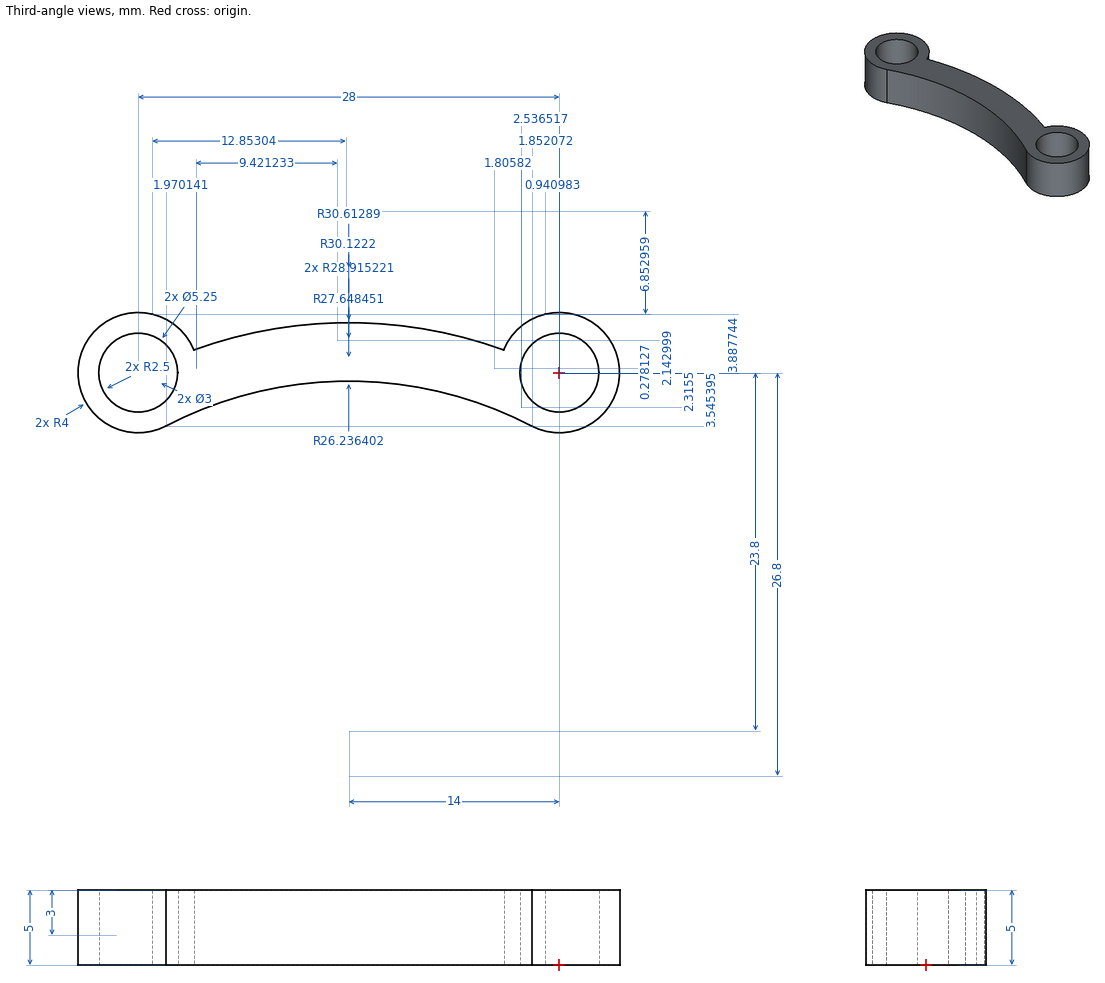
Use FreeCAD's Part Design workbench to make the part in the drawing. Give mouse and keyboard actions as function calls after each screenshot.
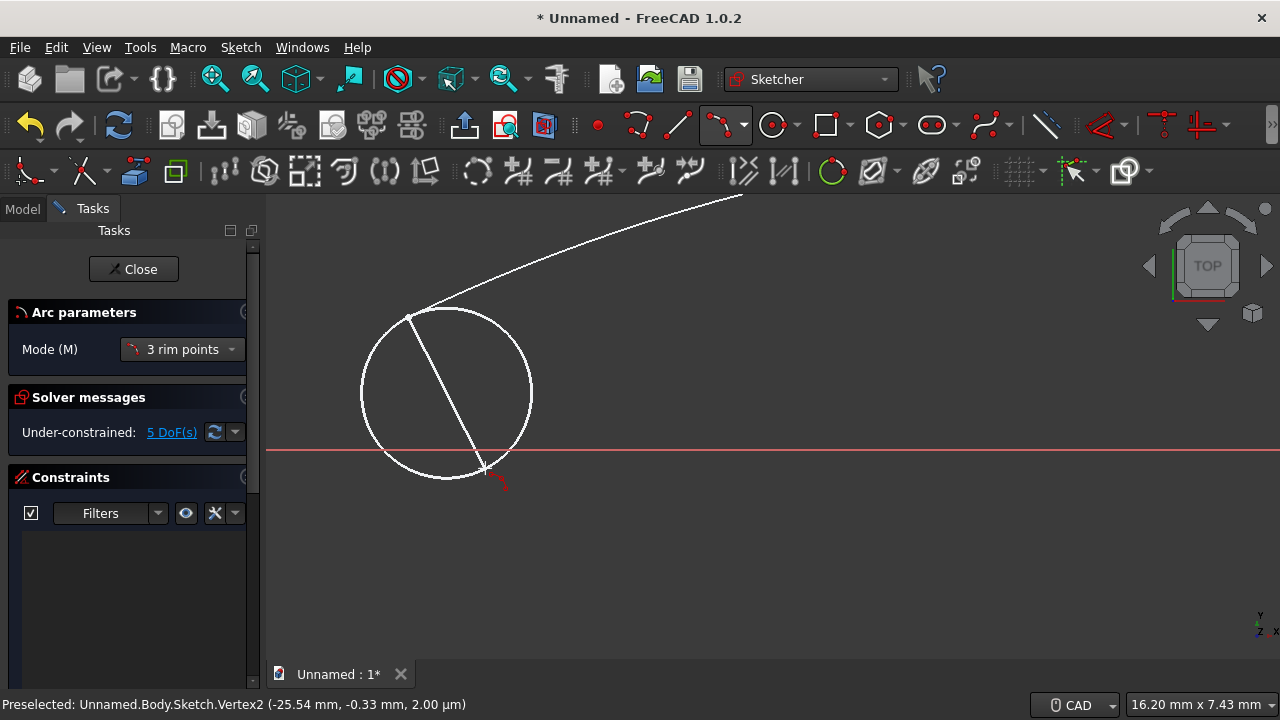
scroll(488, 470, down, 6)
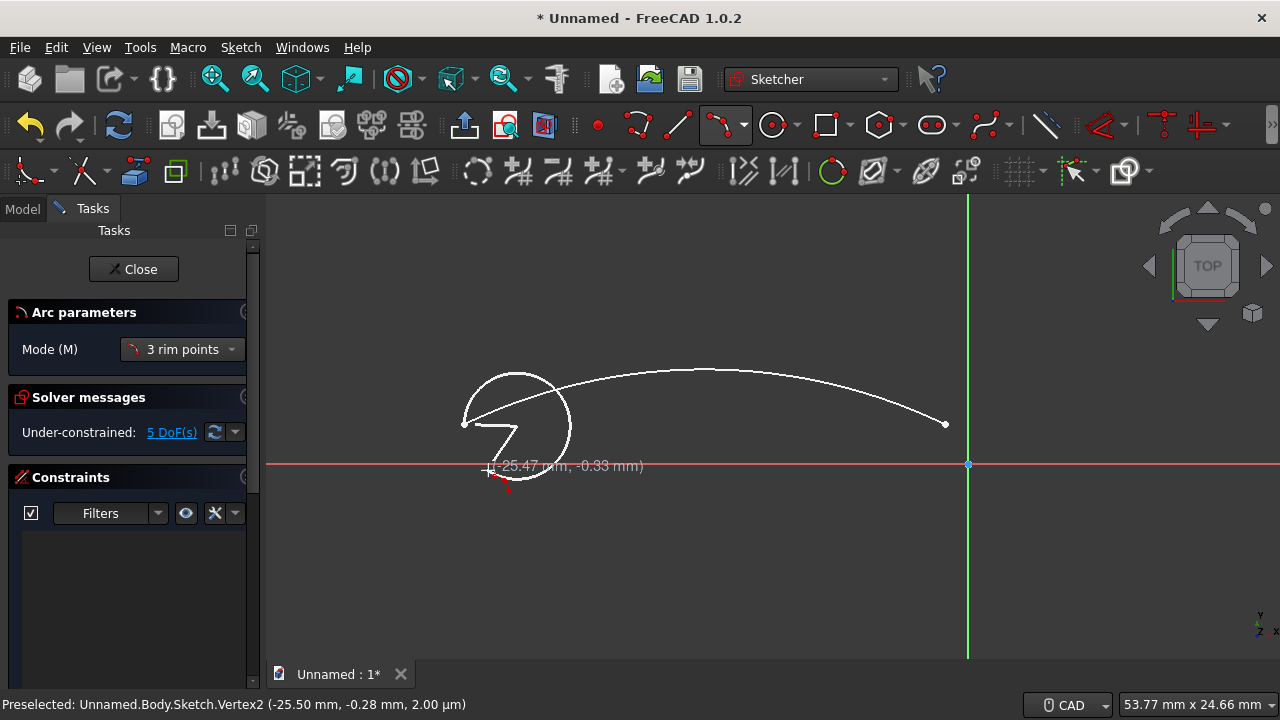
click(398, 486)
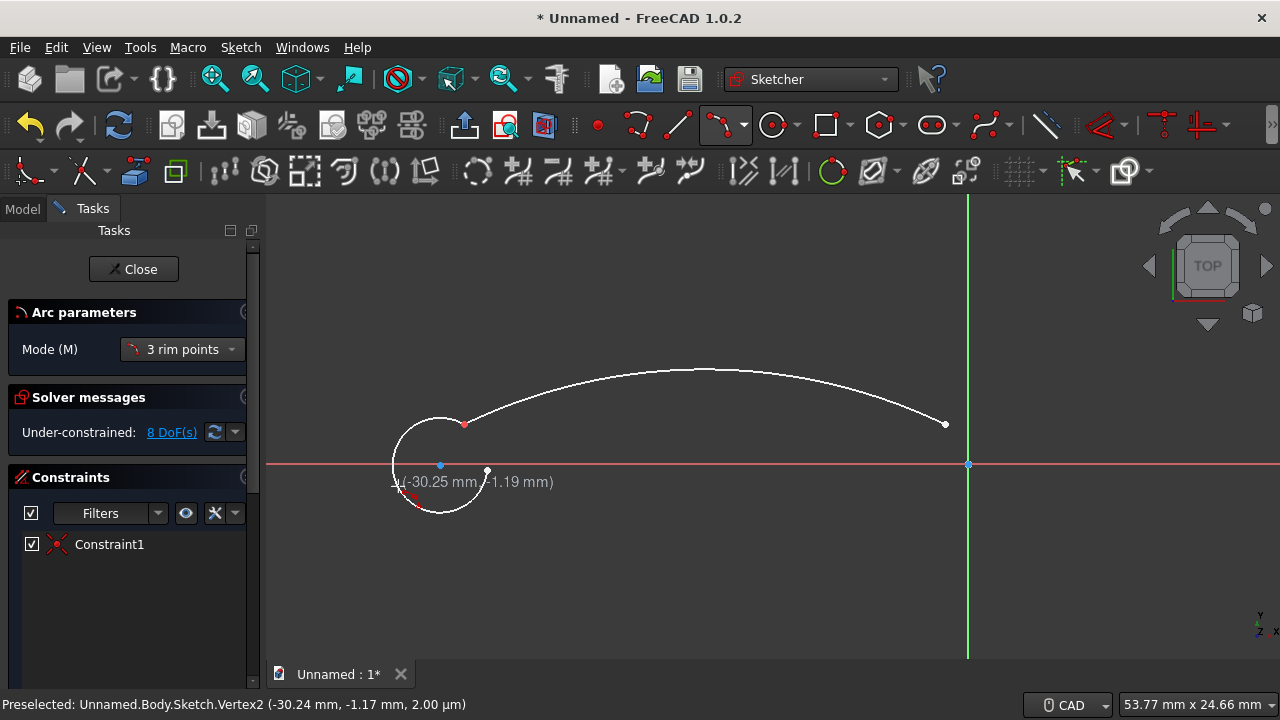
scroll(487, 470, up, 6)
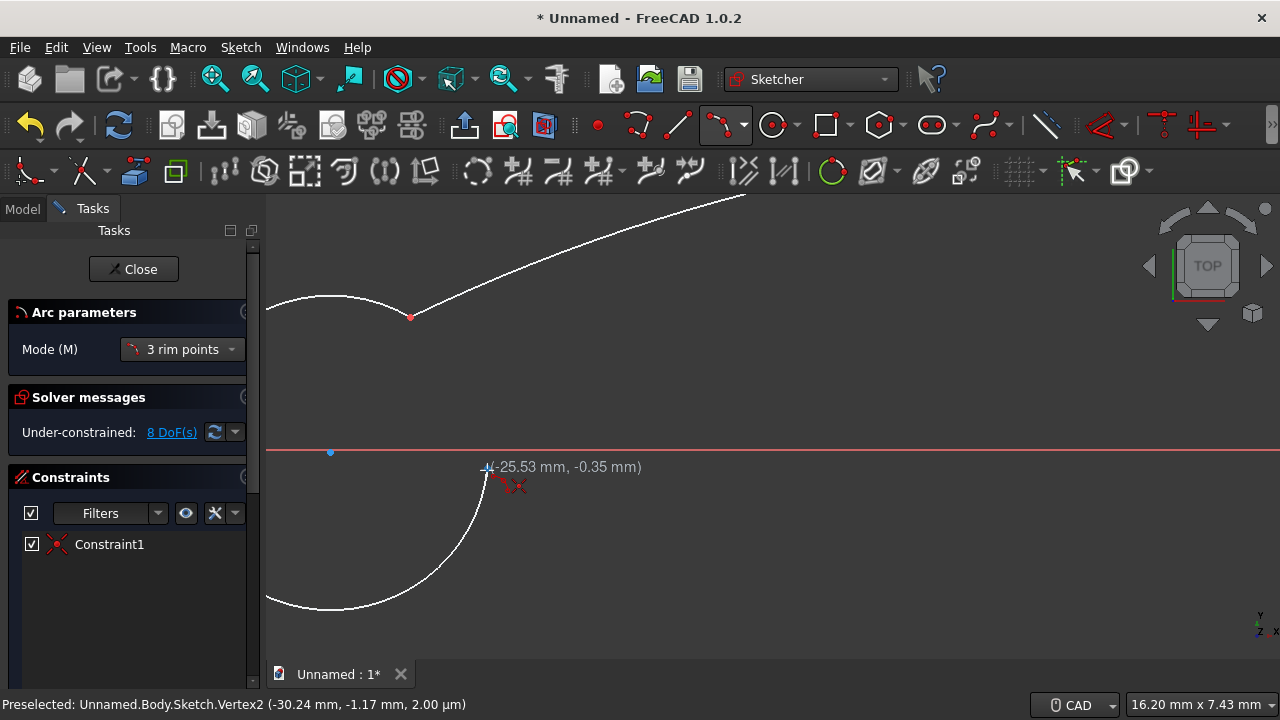
click(487, 469)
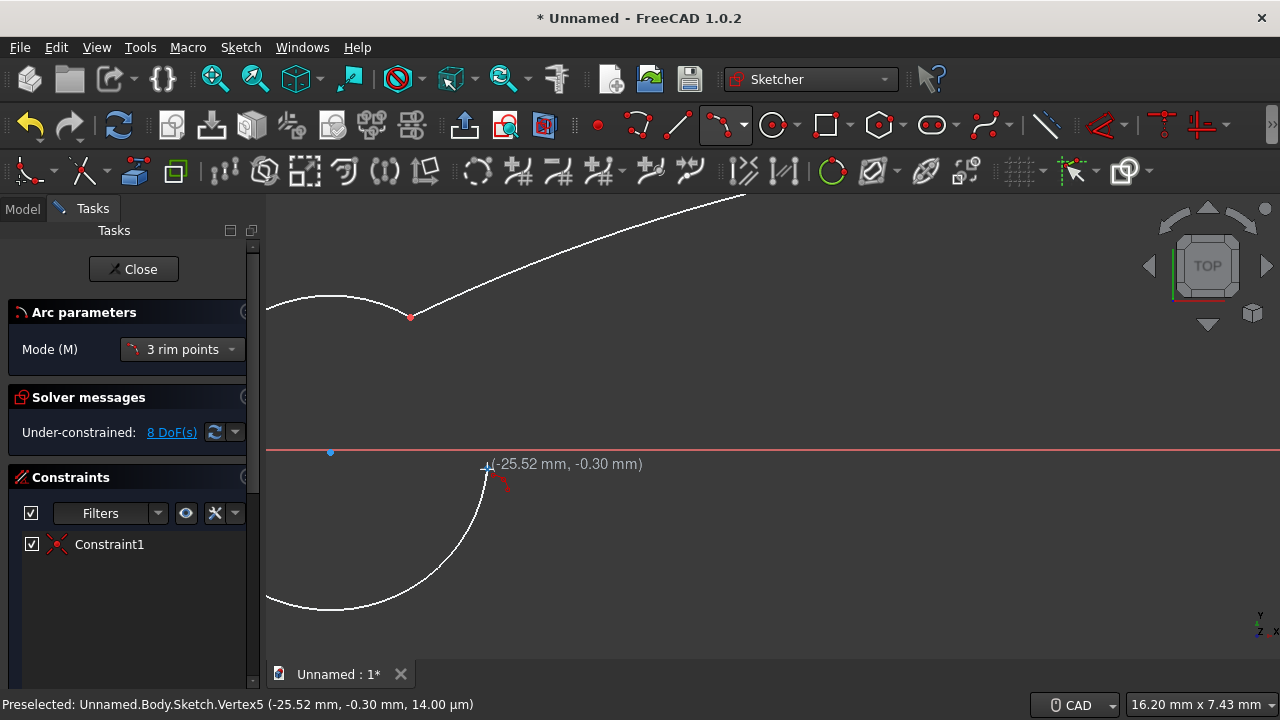
scroll(487, 470, down, 6)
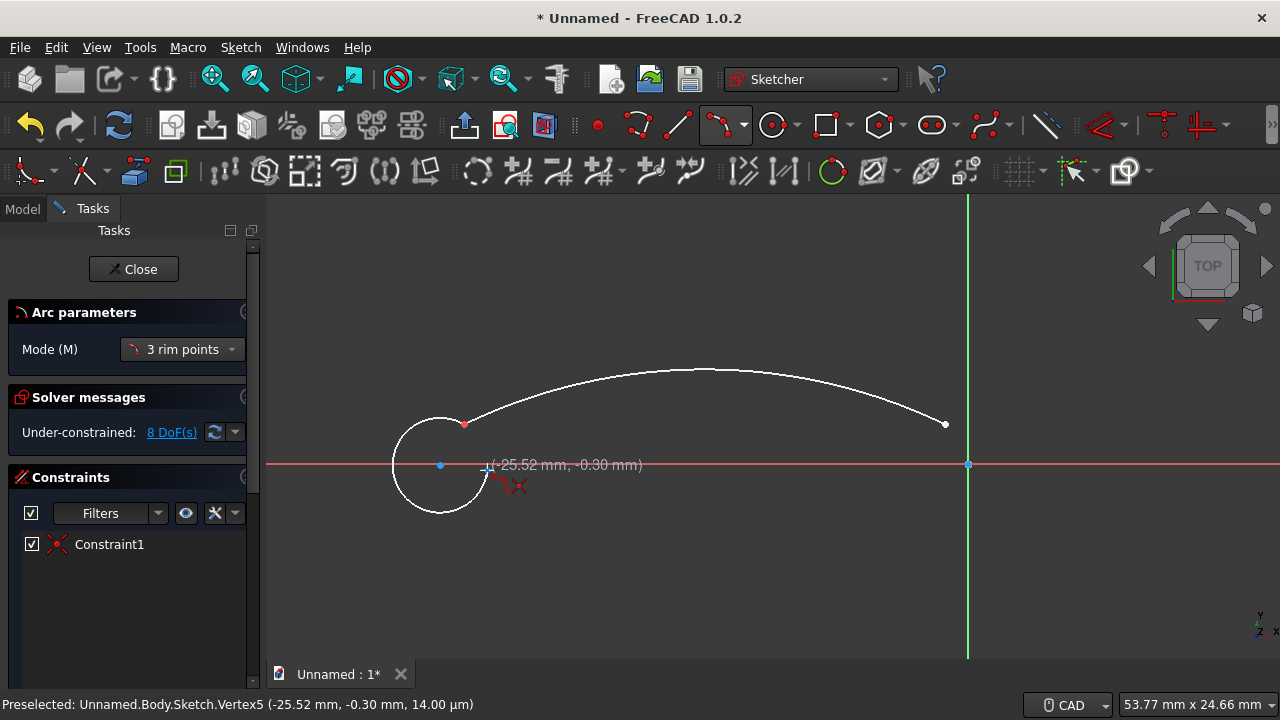
scroll(922, 470, up, 6)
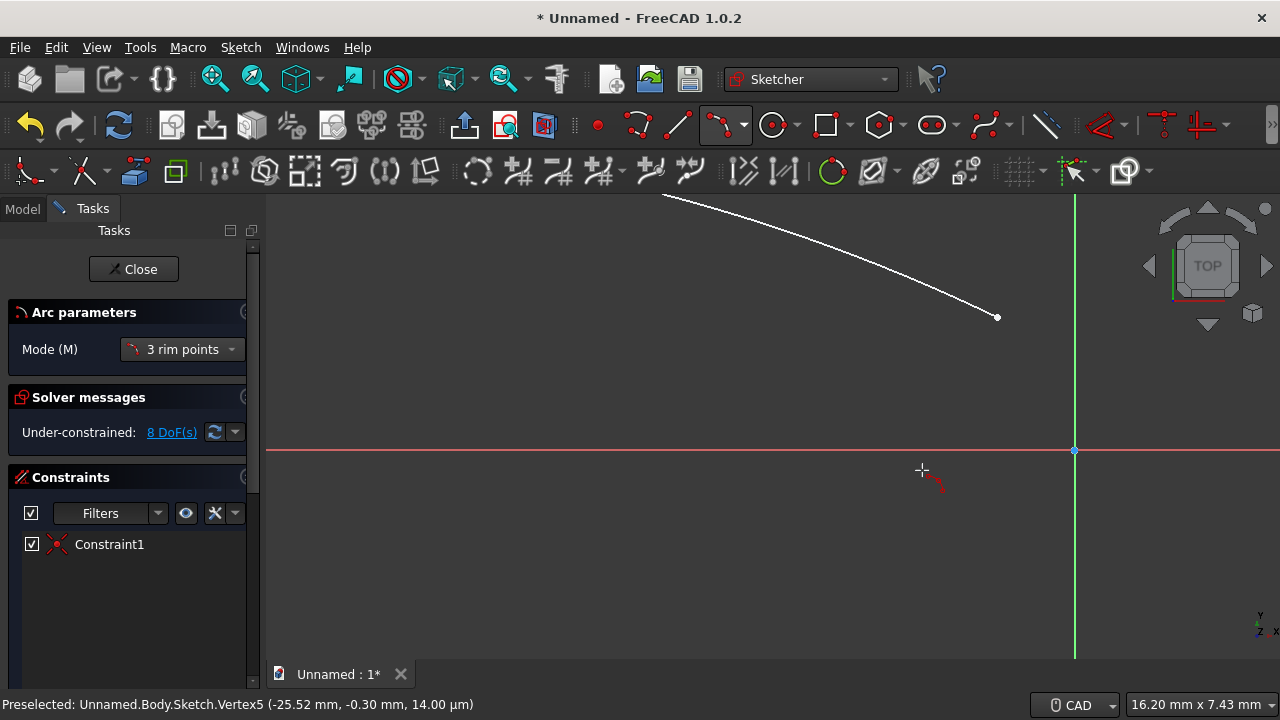
click(919, 468)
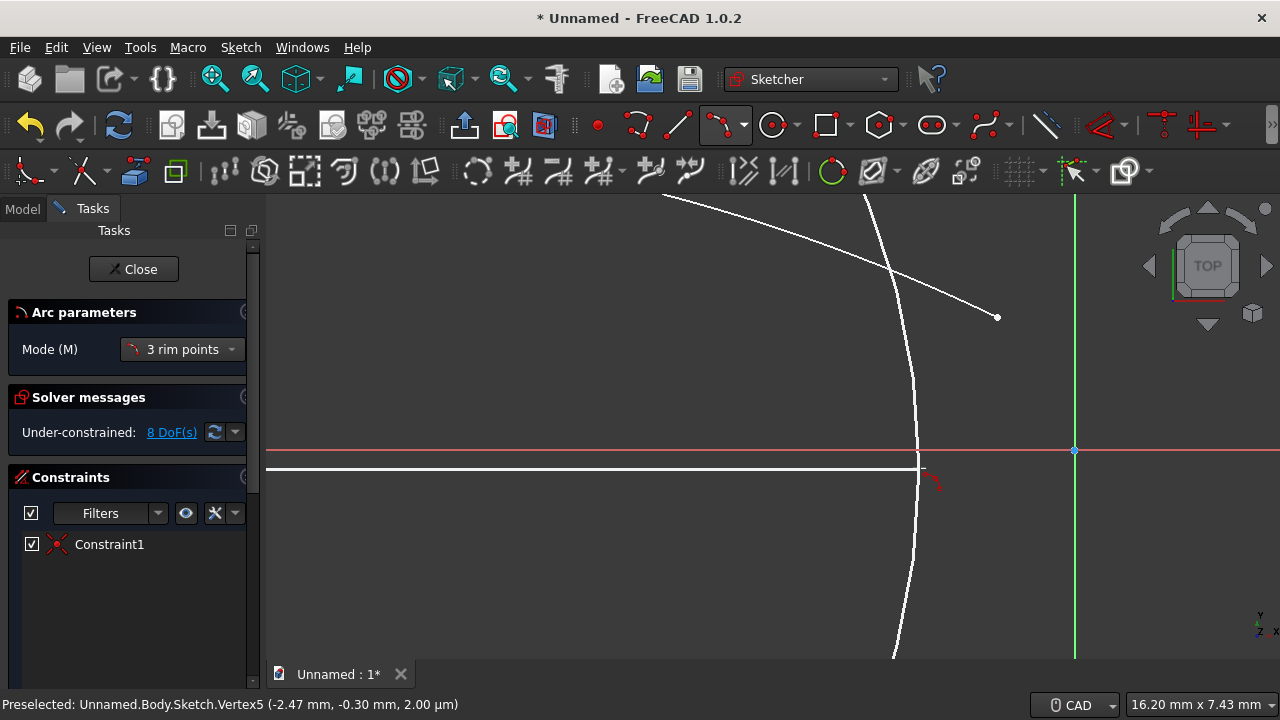
scroll(923, 470, down, 6)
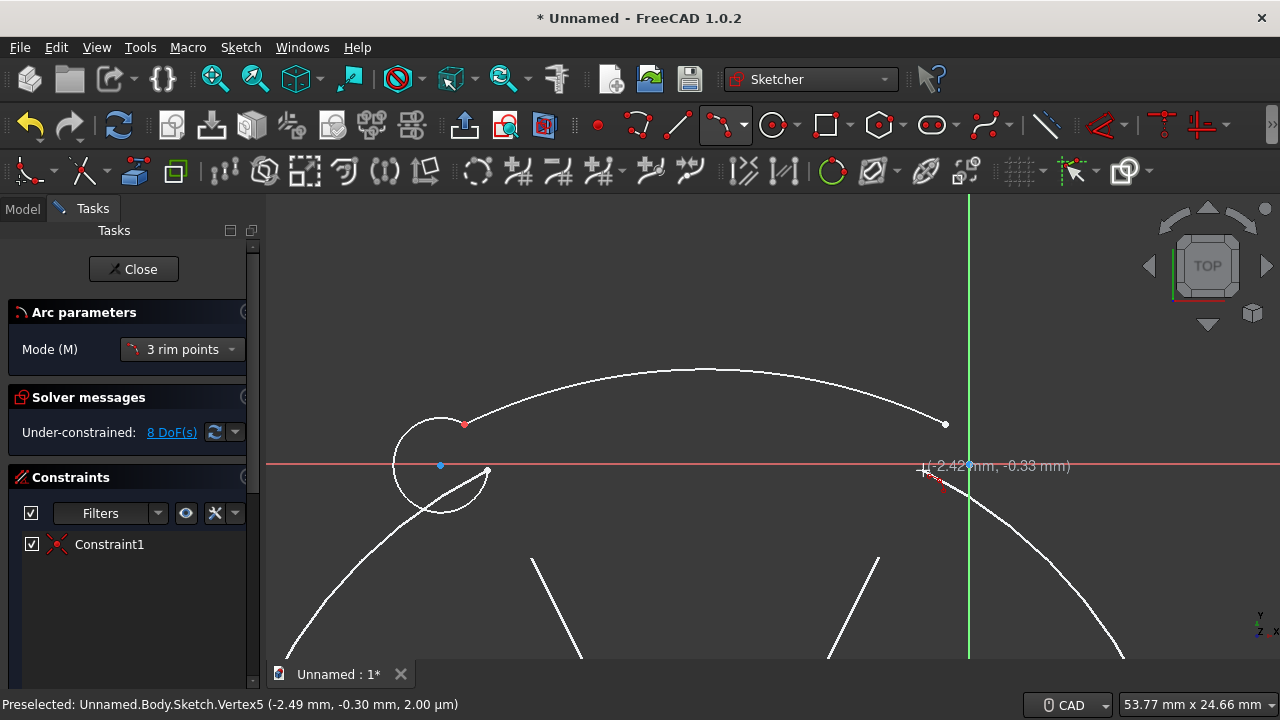
click(705, 425)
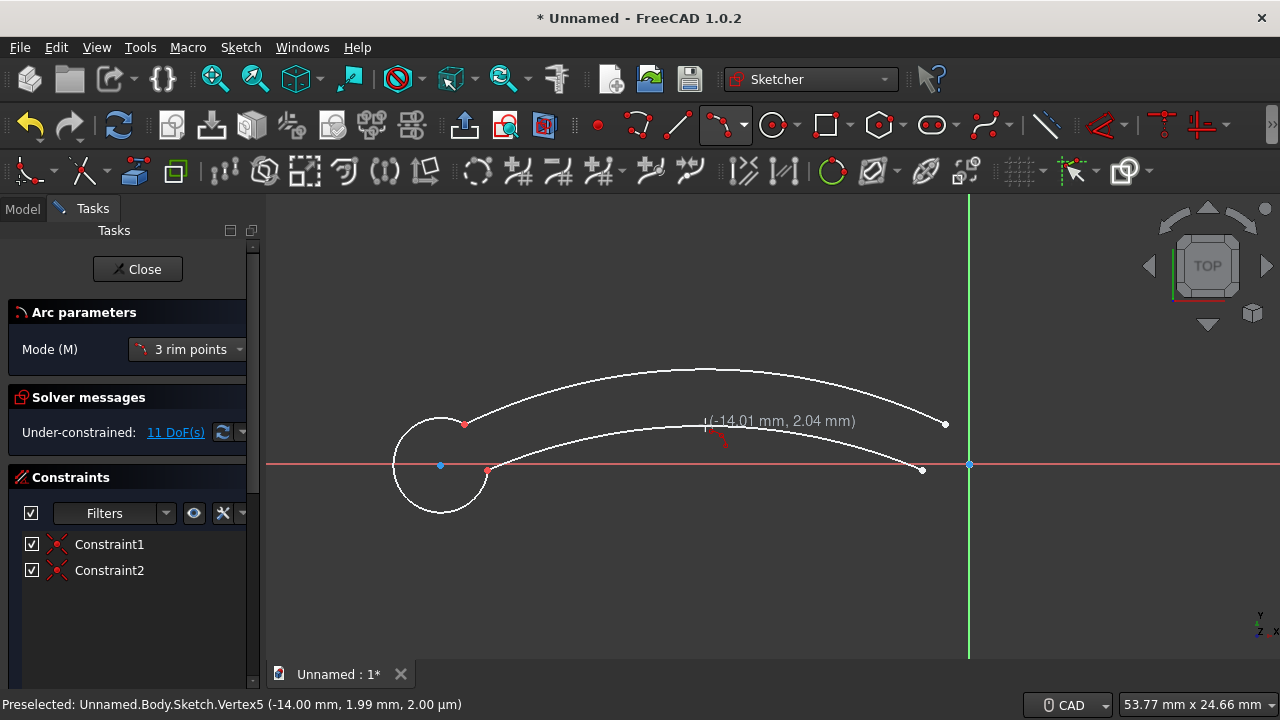
scroll(922, 470, up, 6)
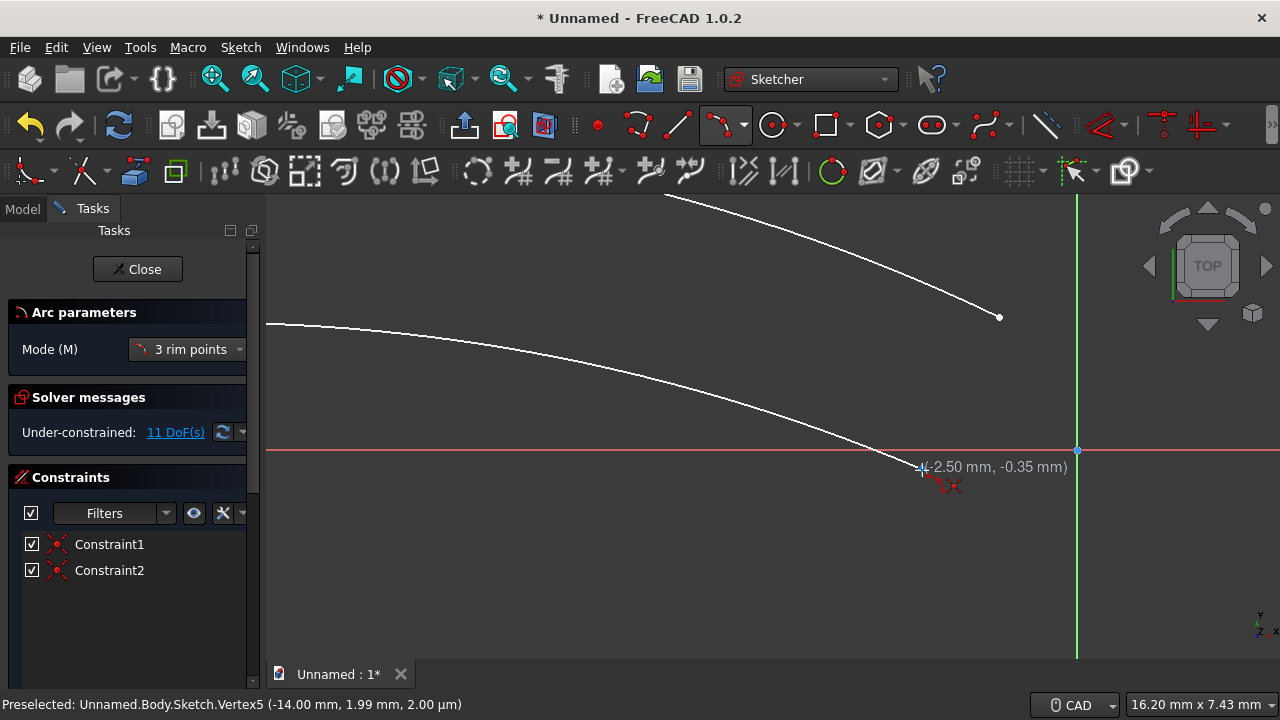
click(921, 469)
click(1000, 317)